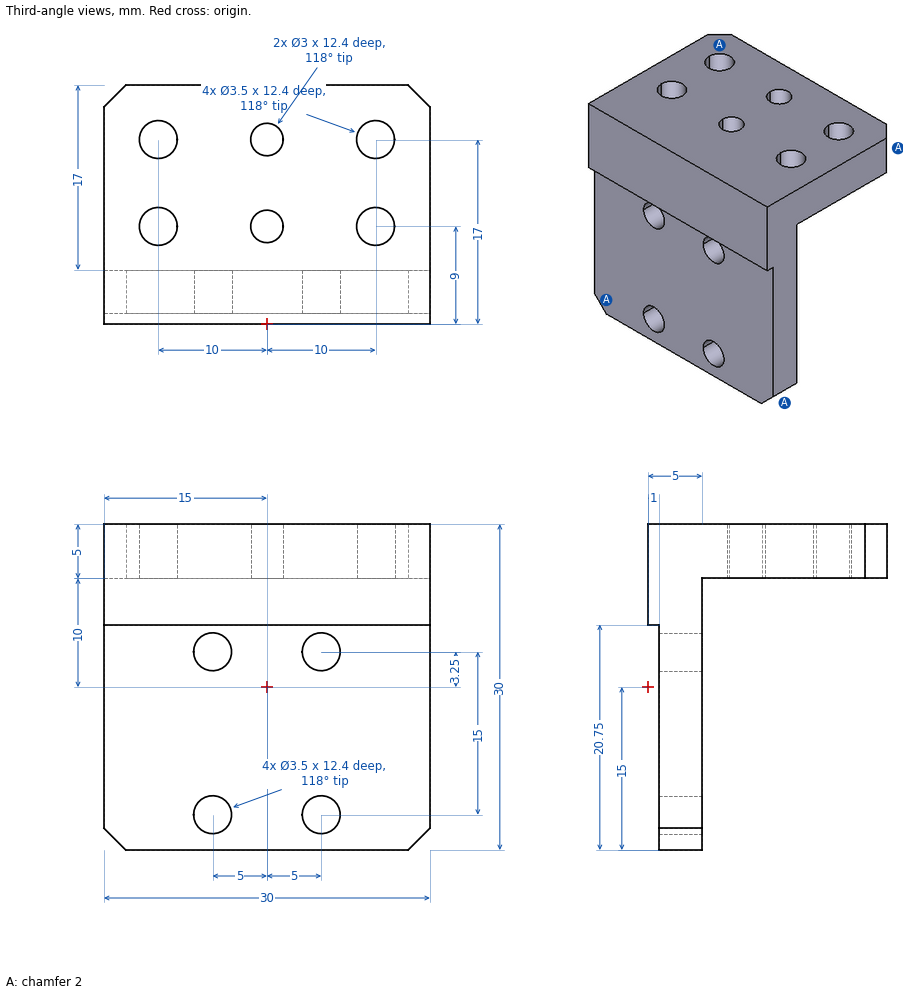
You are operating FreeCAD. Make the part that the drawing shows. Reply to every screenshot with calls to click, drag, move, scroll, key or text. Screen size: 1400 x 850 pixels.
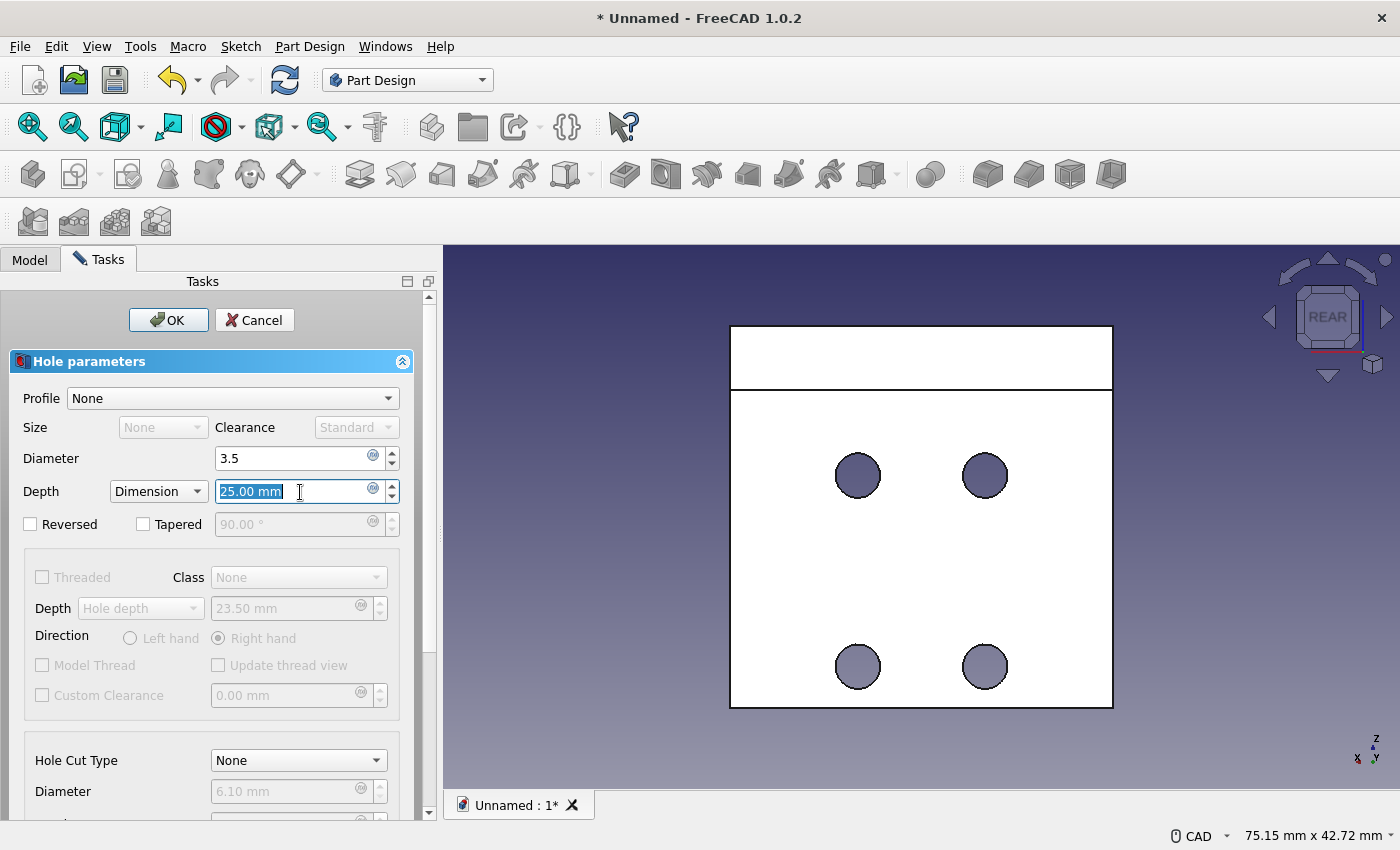
text(12.4)
key(Tab)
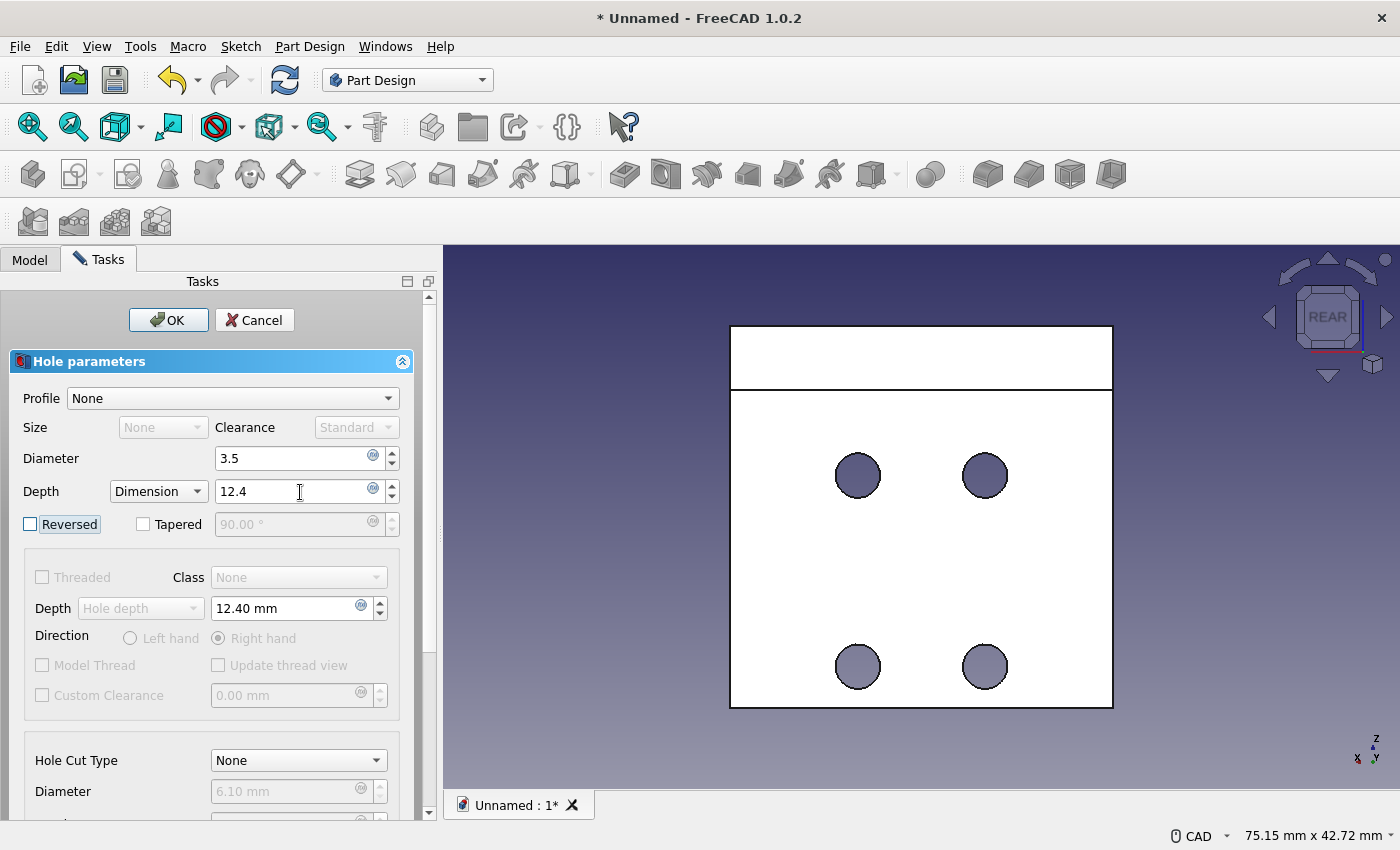
click(169, 320)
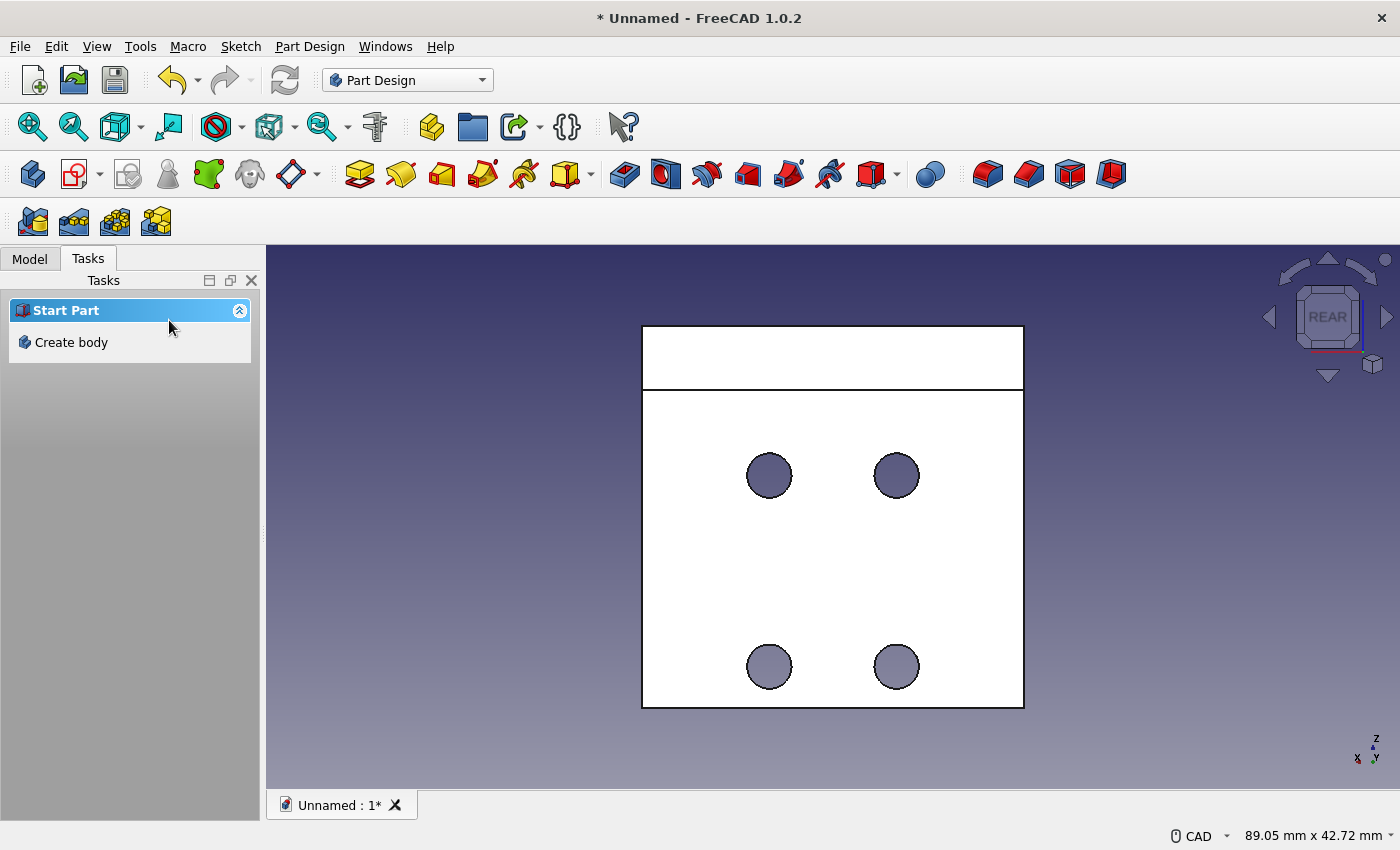
key(6)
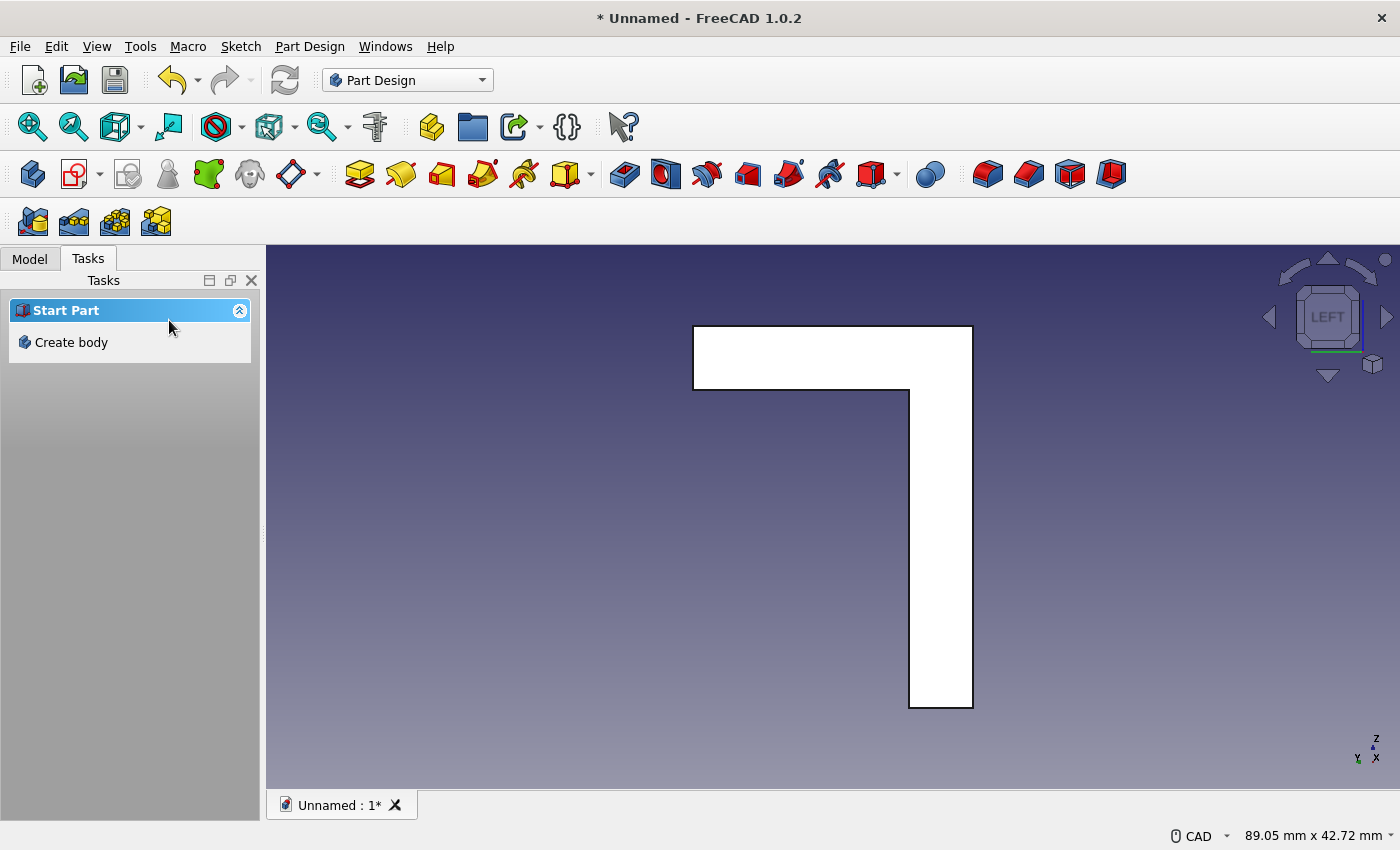
click(833, 352)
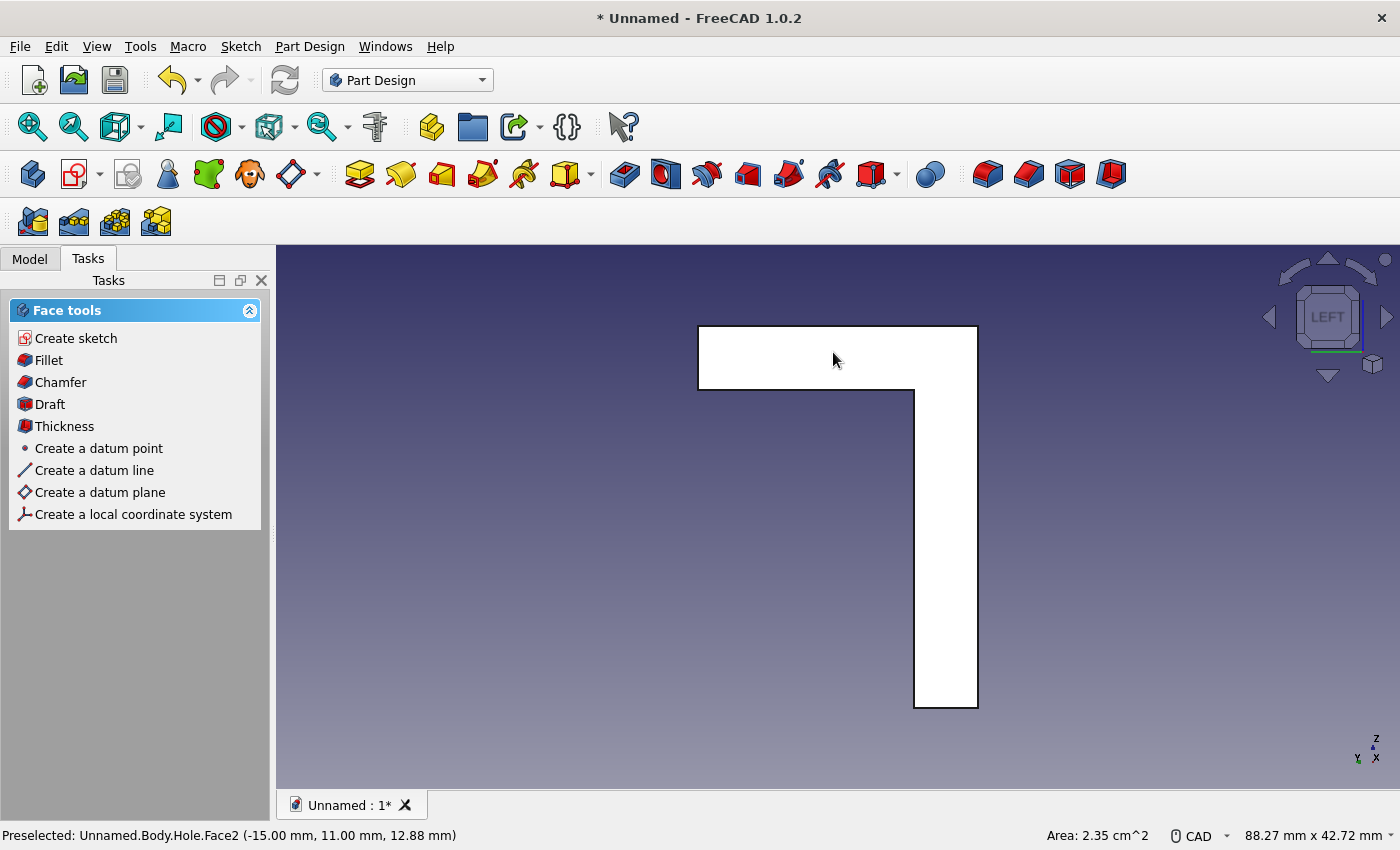
click(74, 174)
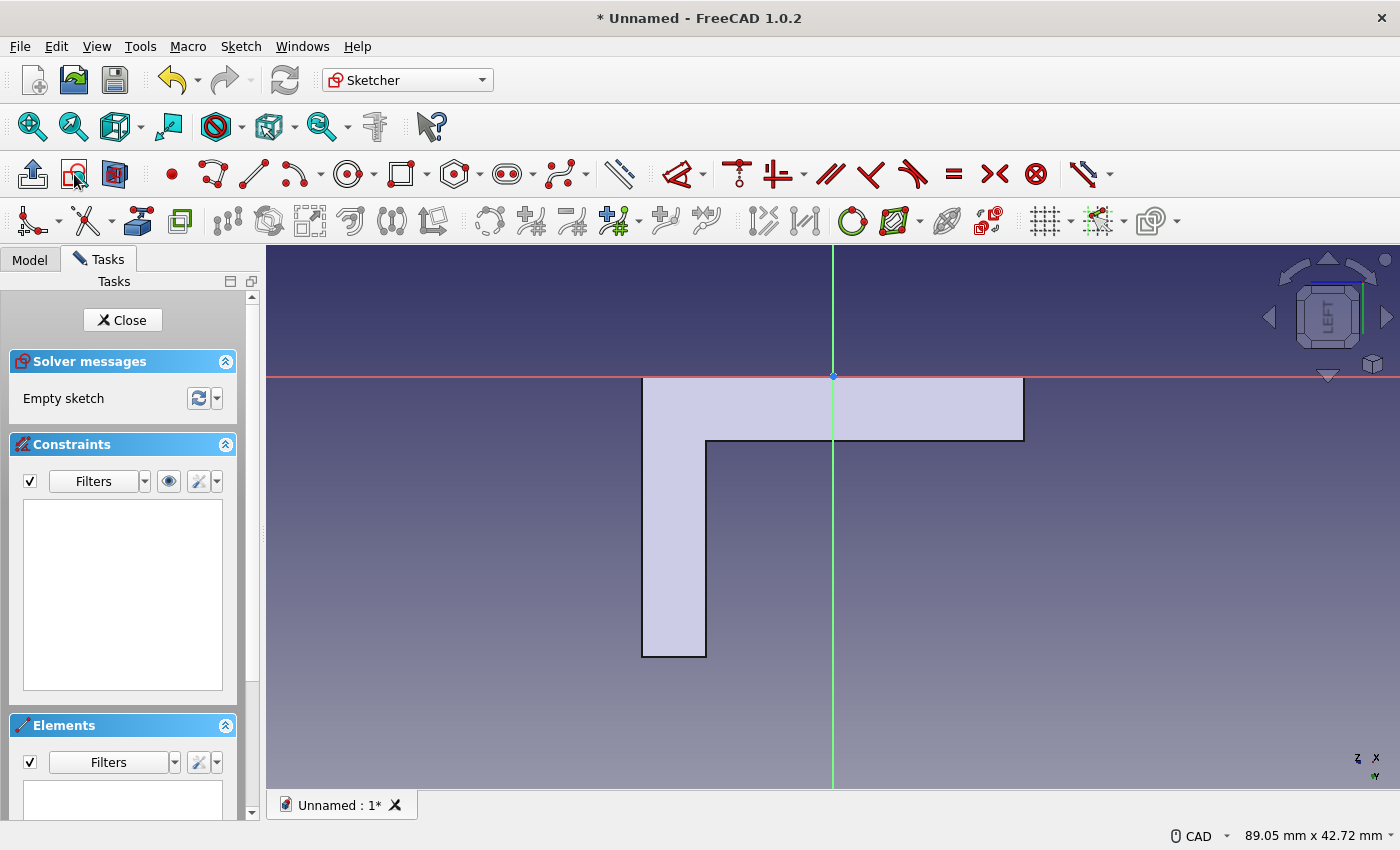
scroll(966, 305, up, 5)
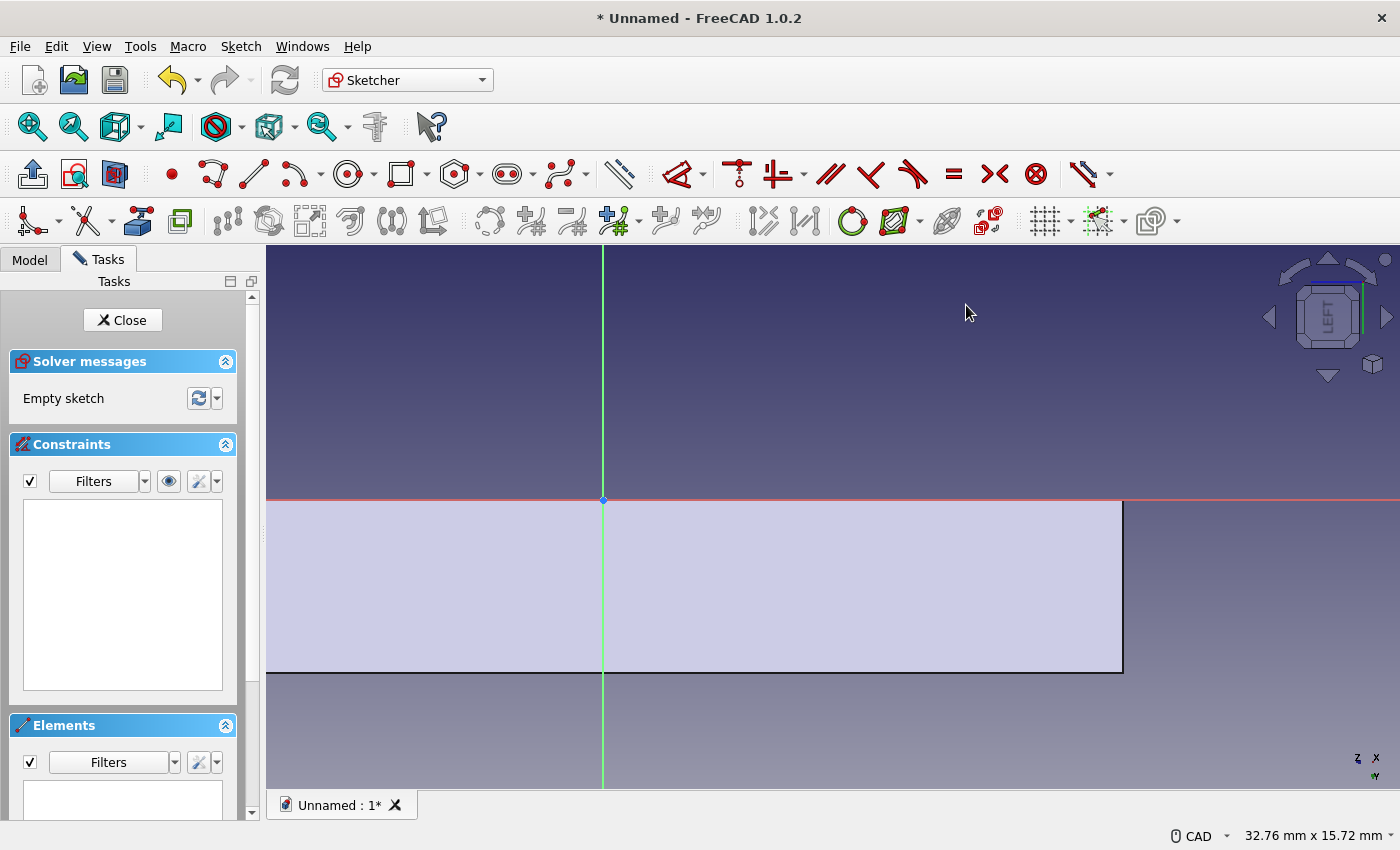
key(g)
key(r)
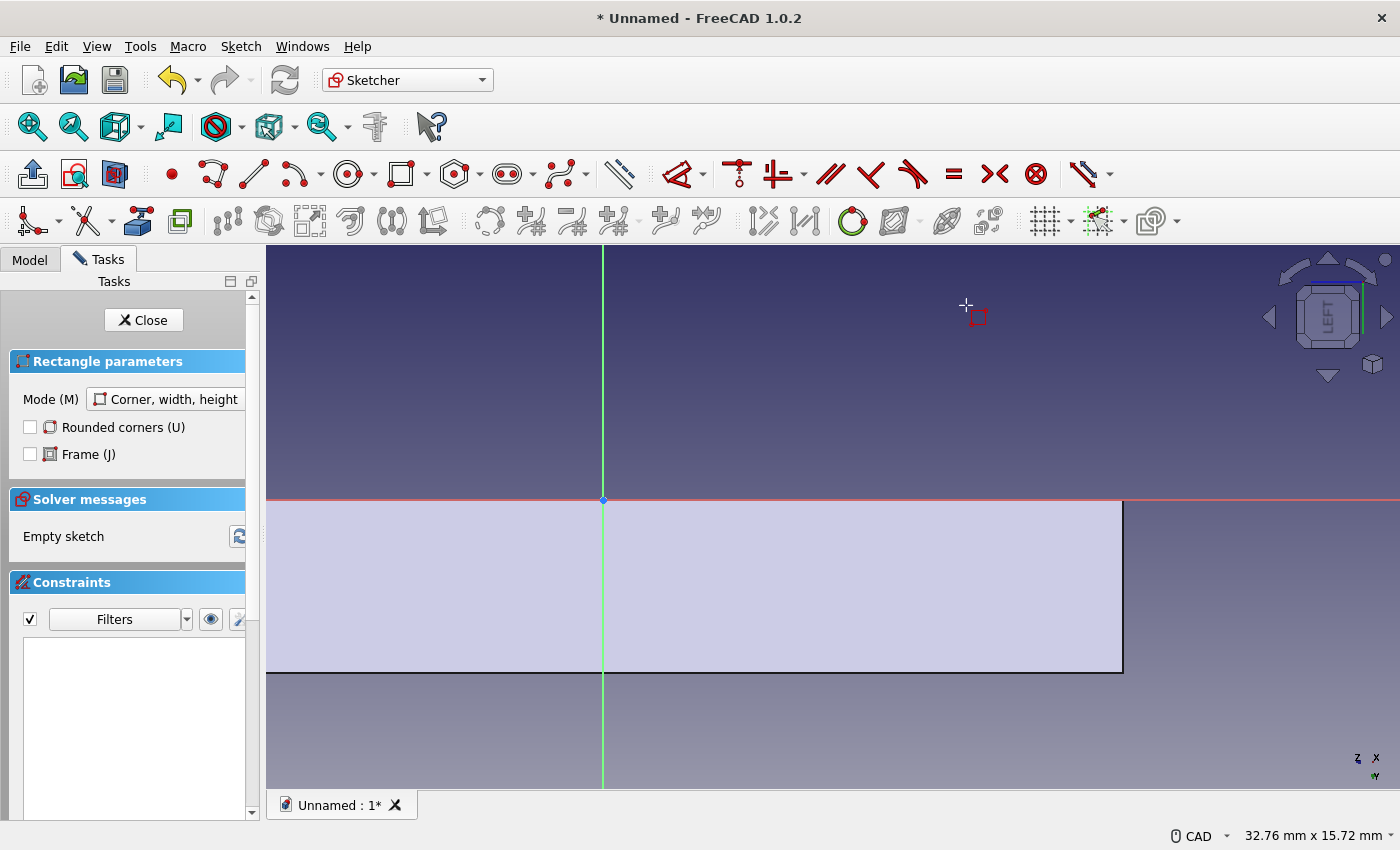
click(404, 500)
click(1123, 535)
key(Escape)